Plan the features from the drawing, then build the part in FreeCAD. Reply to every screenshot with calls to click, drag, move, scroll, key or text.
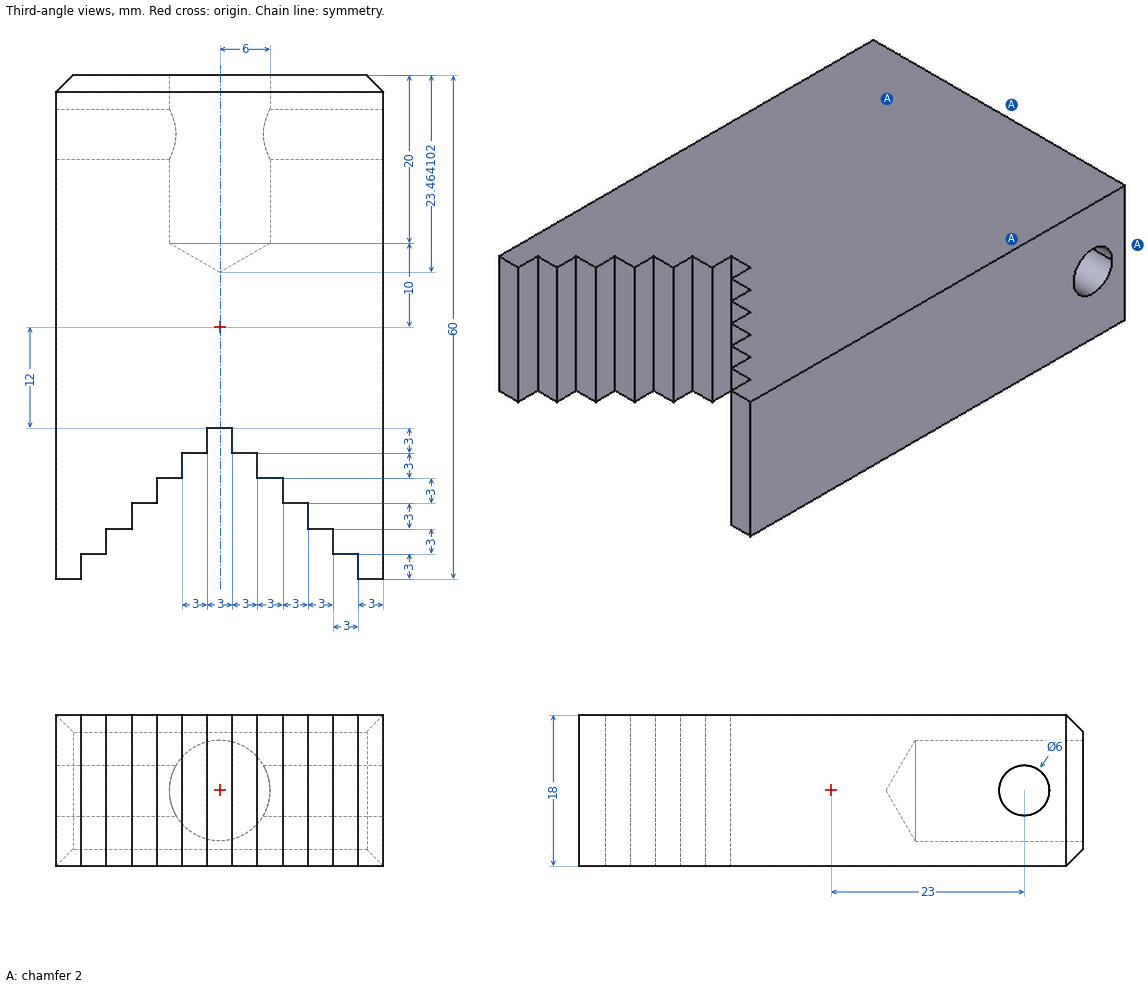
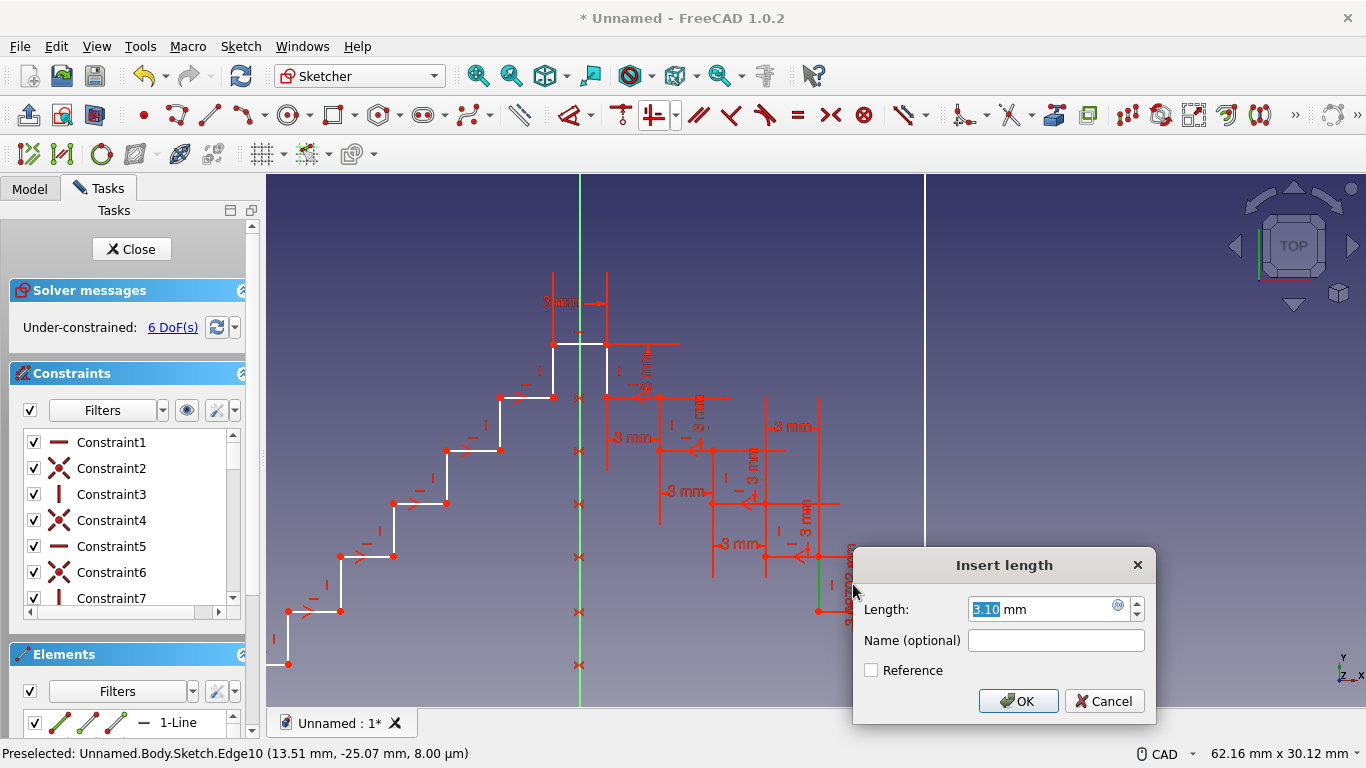
text(3)
key(Return)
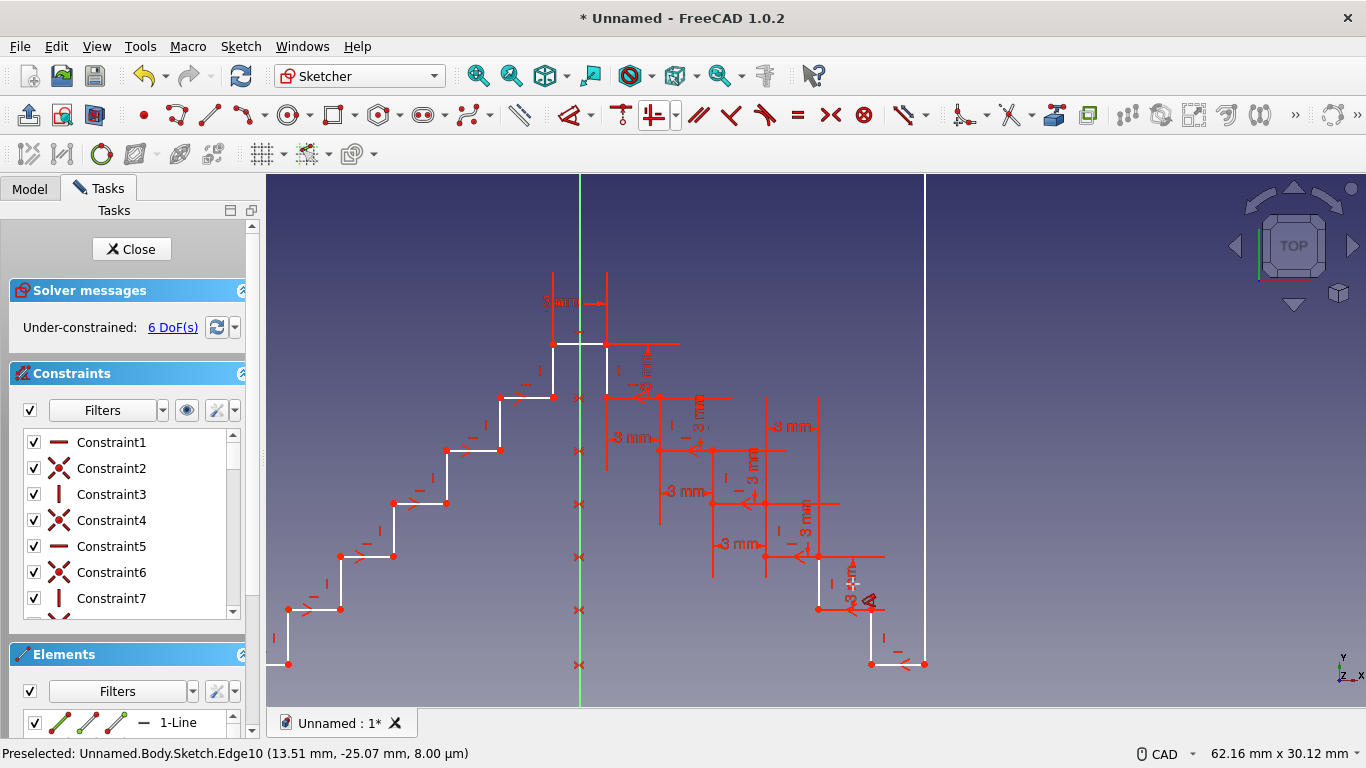
click(835, 610)
click(845, 644)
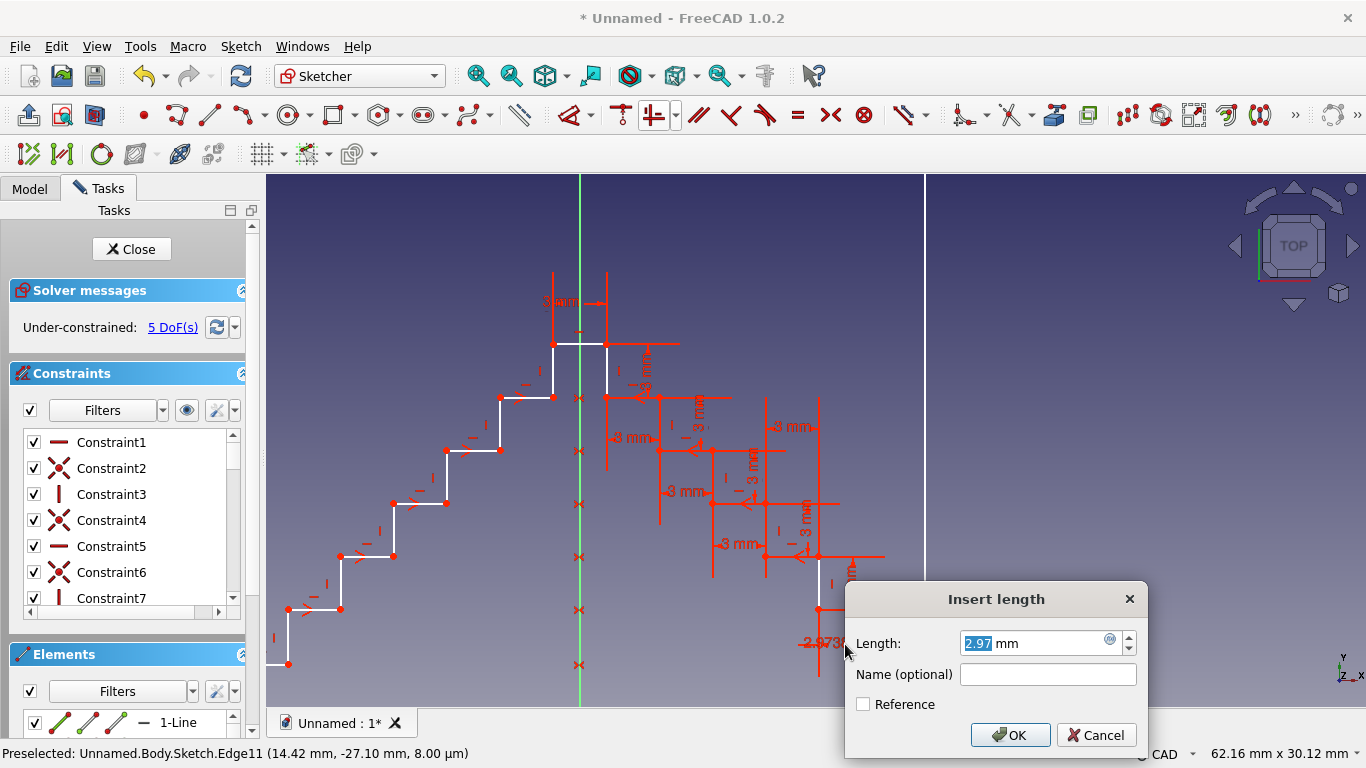
text(3)
key(Return)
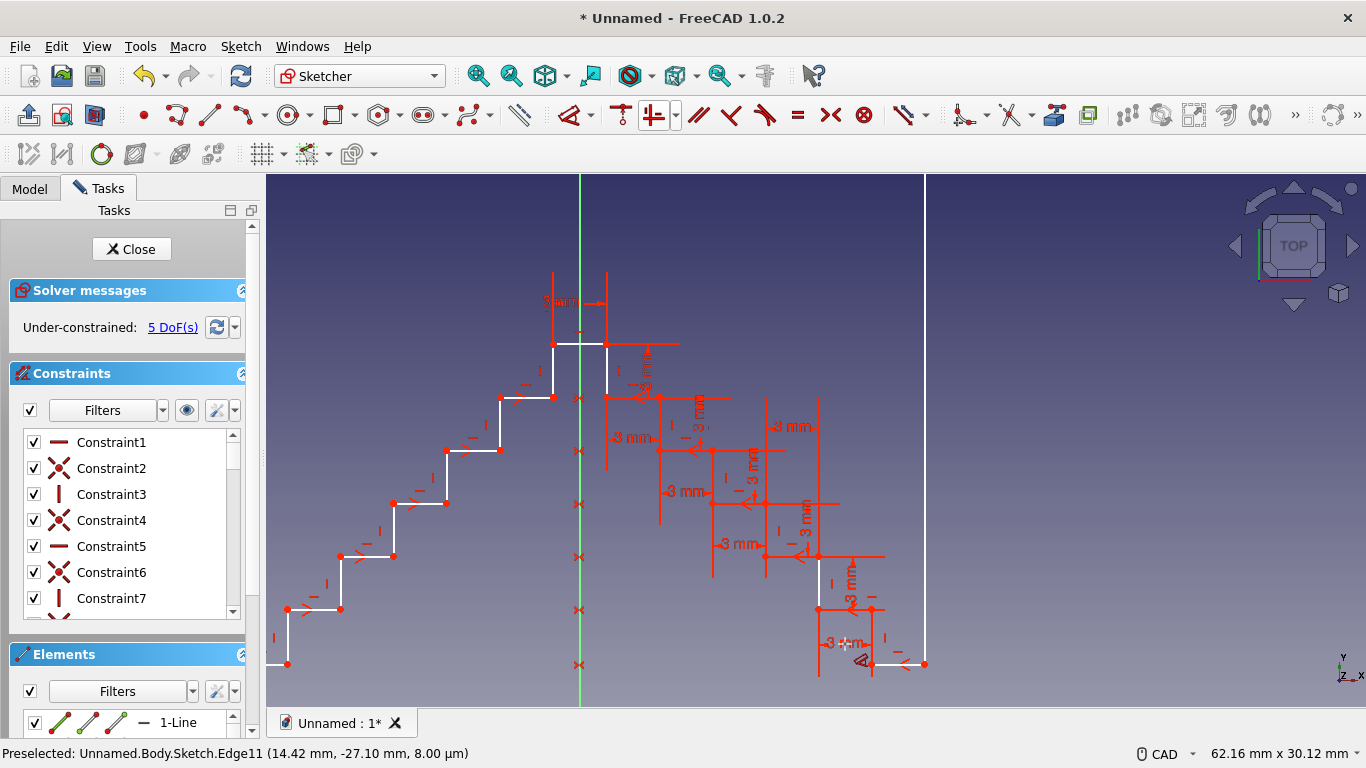
click(872, 626)
click(906, 618)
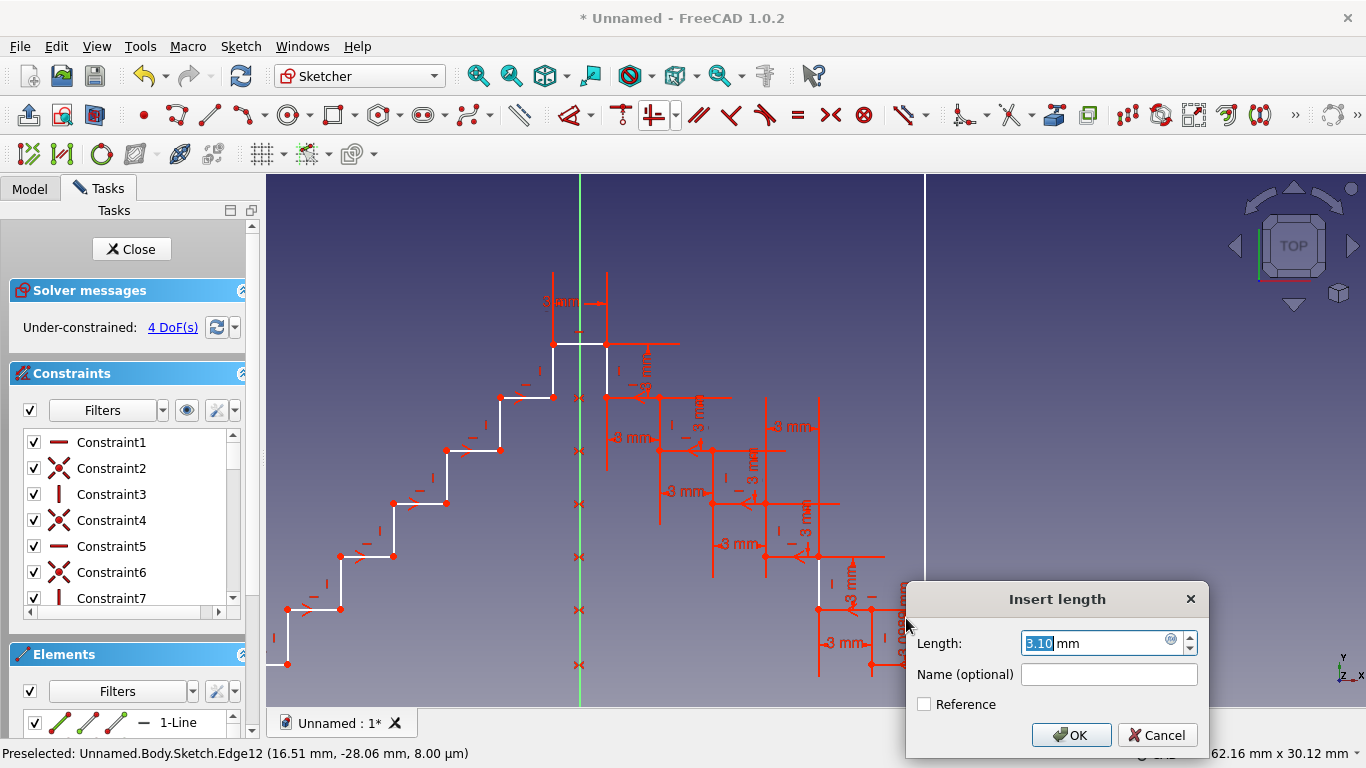
text(3)
key(Return)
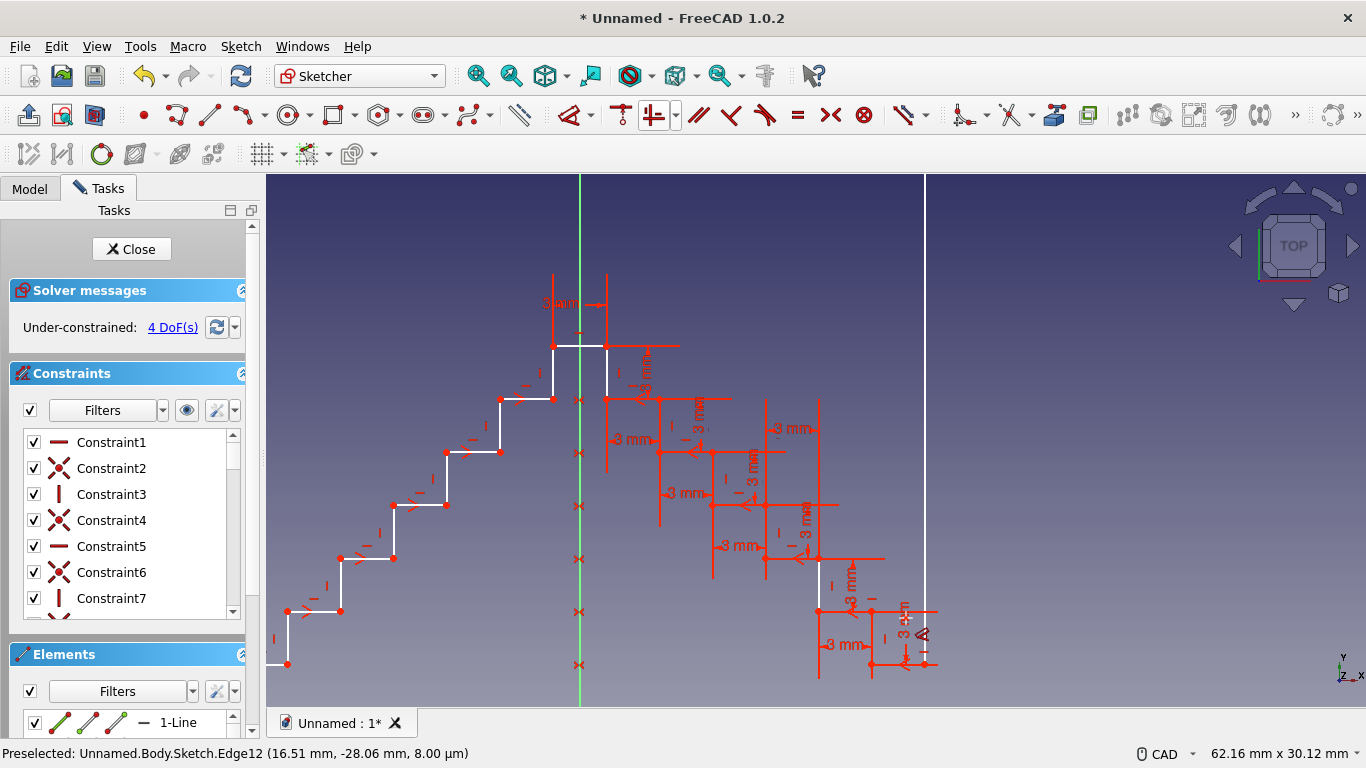
click(888, 665)
click(898, 559)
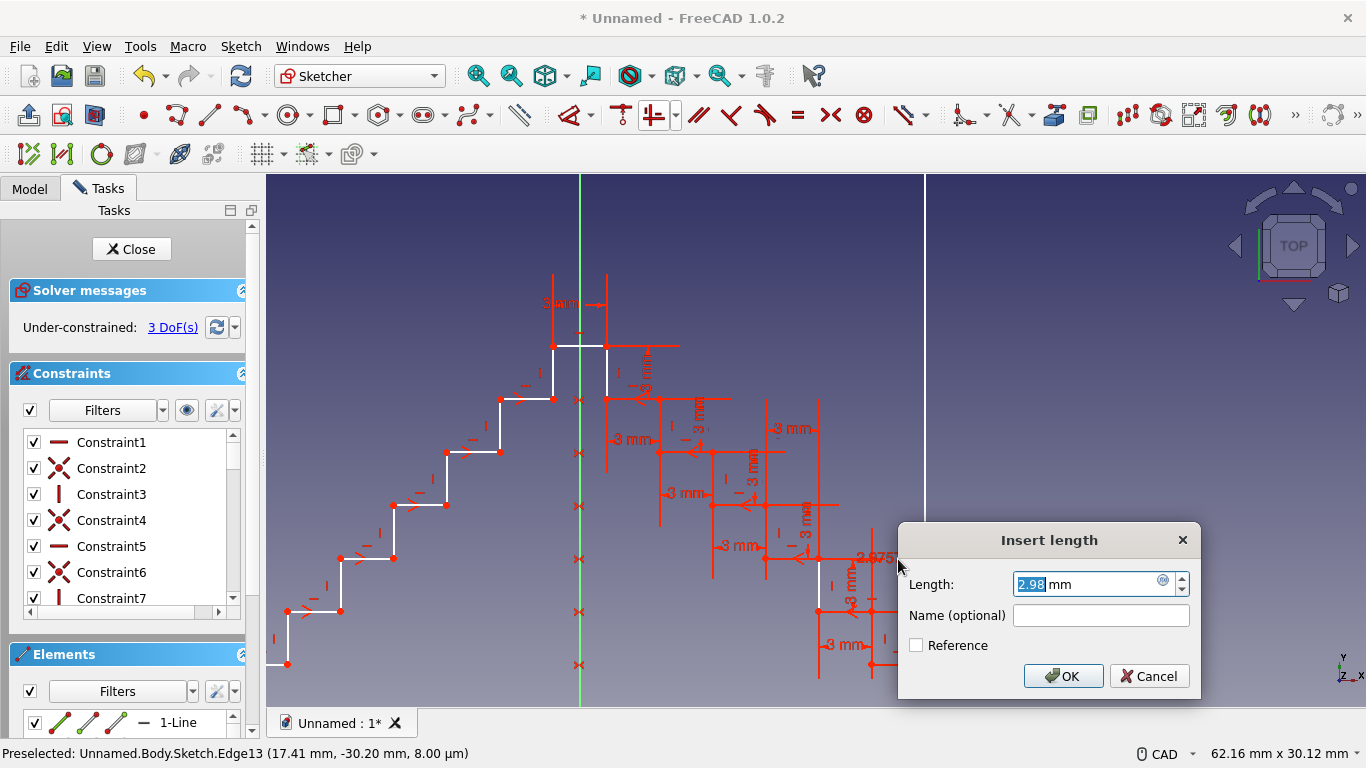
text(3)
key(Return)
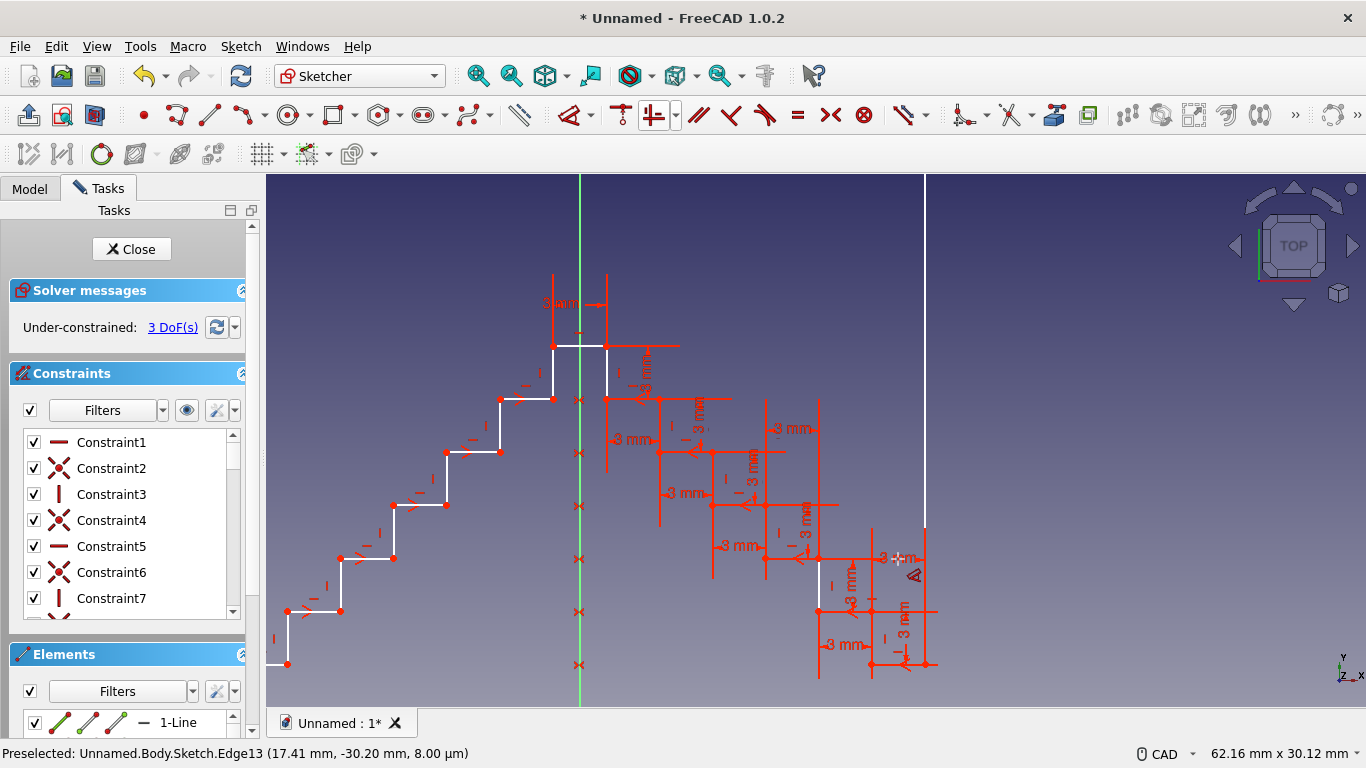
click(516, 399)
click(527, 433)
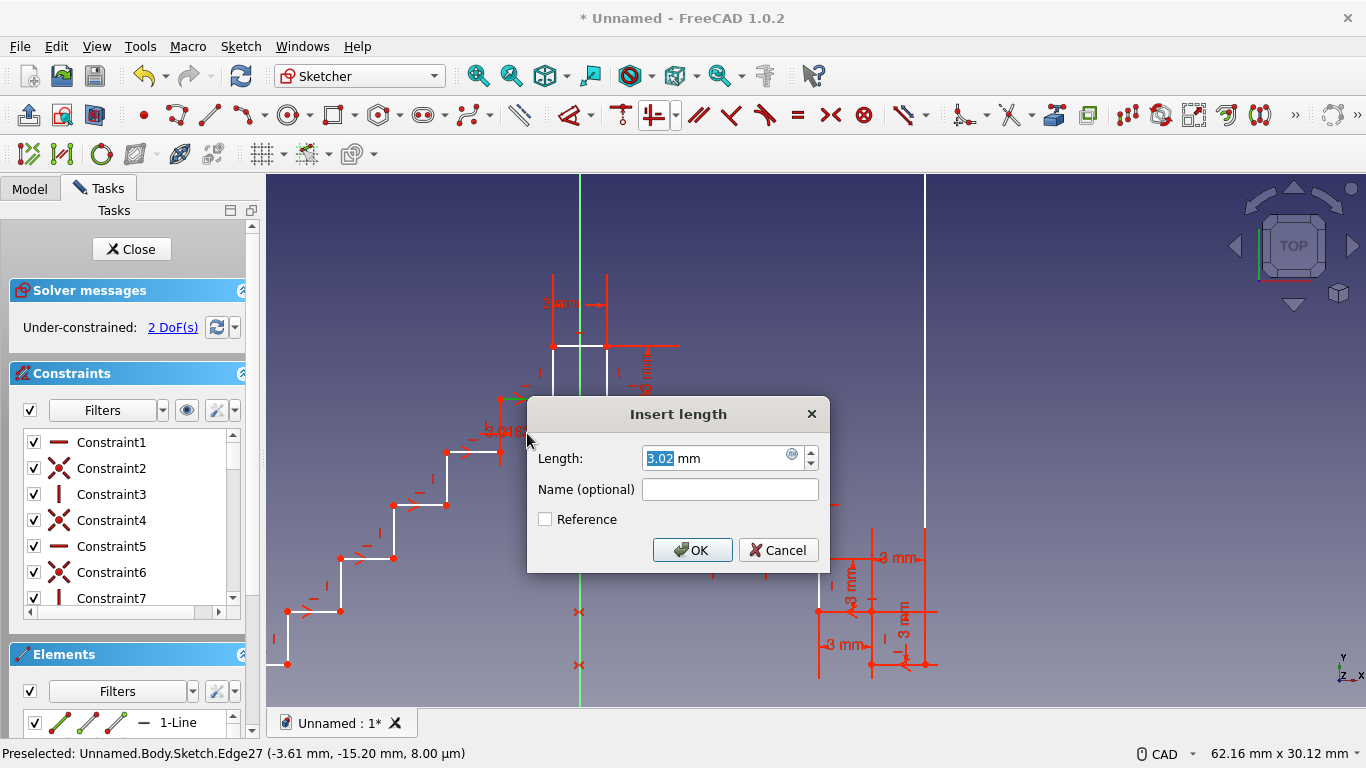
text(3)
key(Return)